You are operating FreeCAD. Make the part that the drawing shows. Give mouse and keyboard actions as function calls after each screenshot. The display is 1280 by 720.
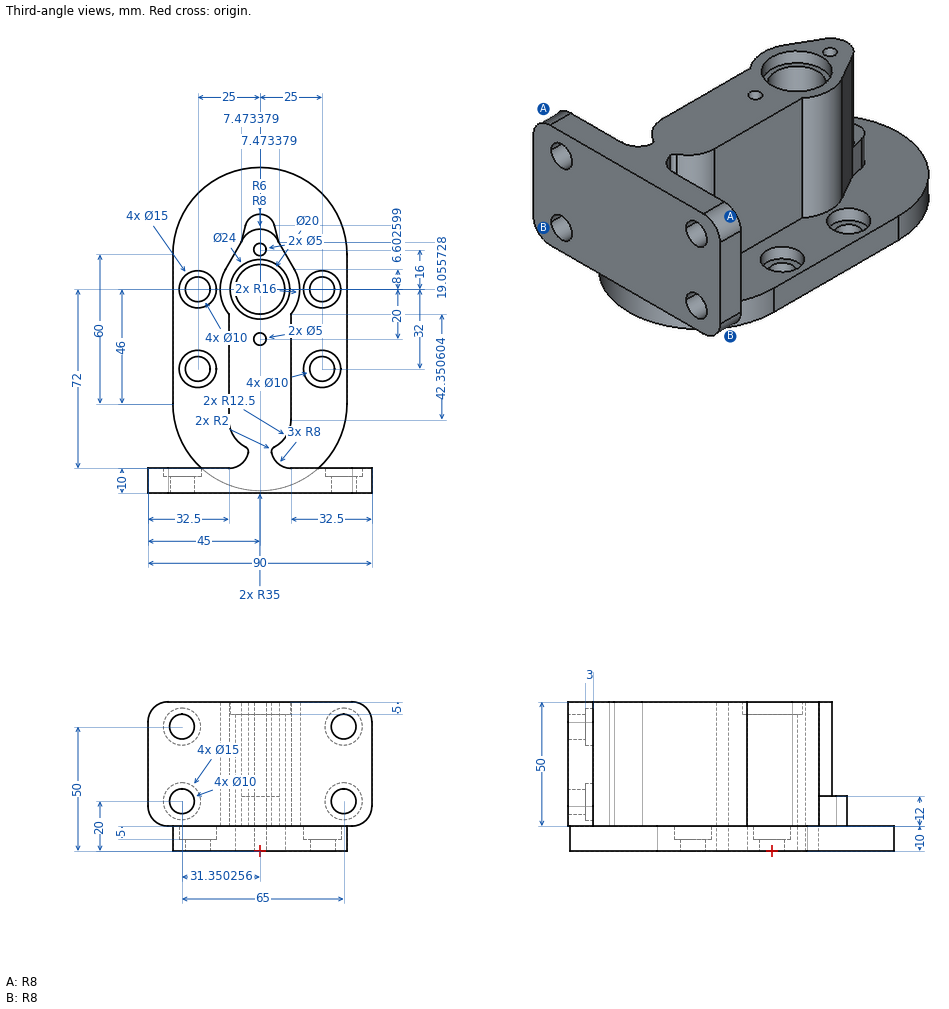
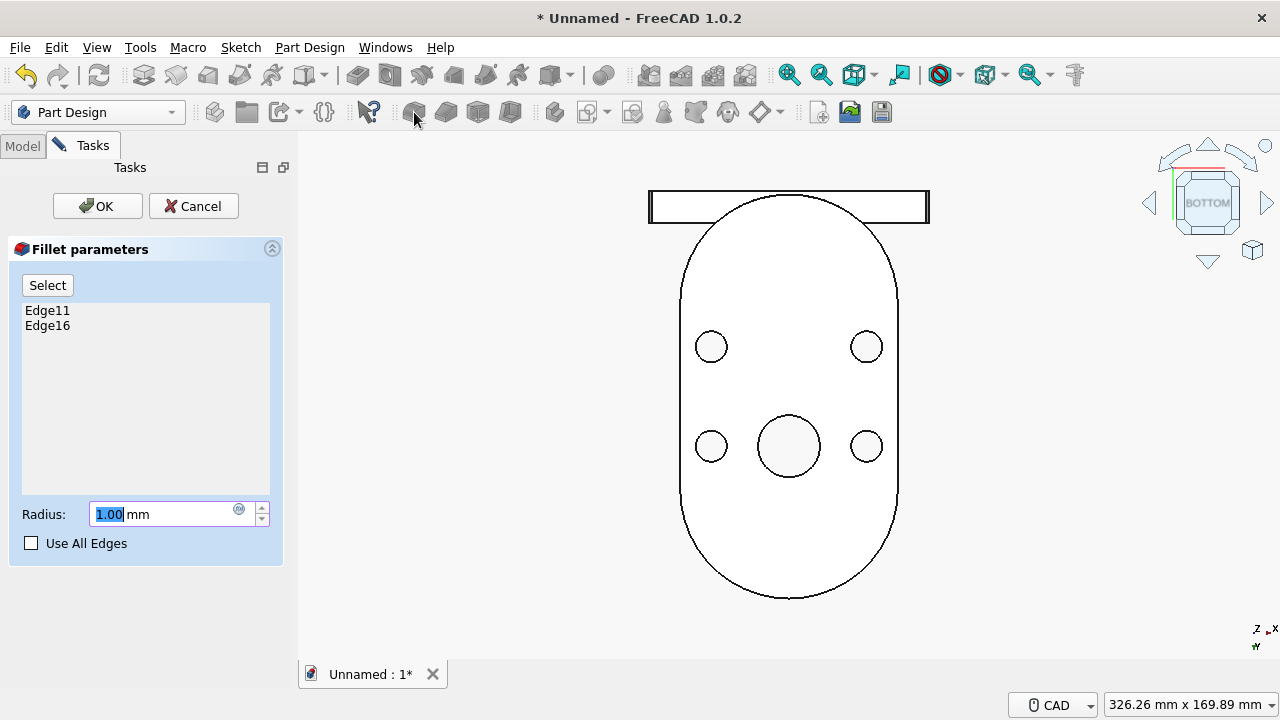
text(8)
key(Tab)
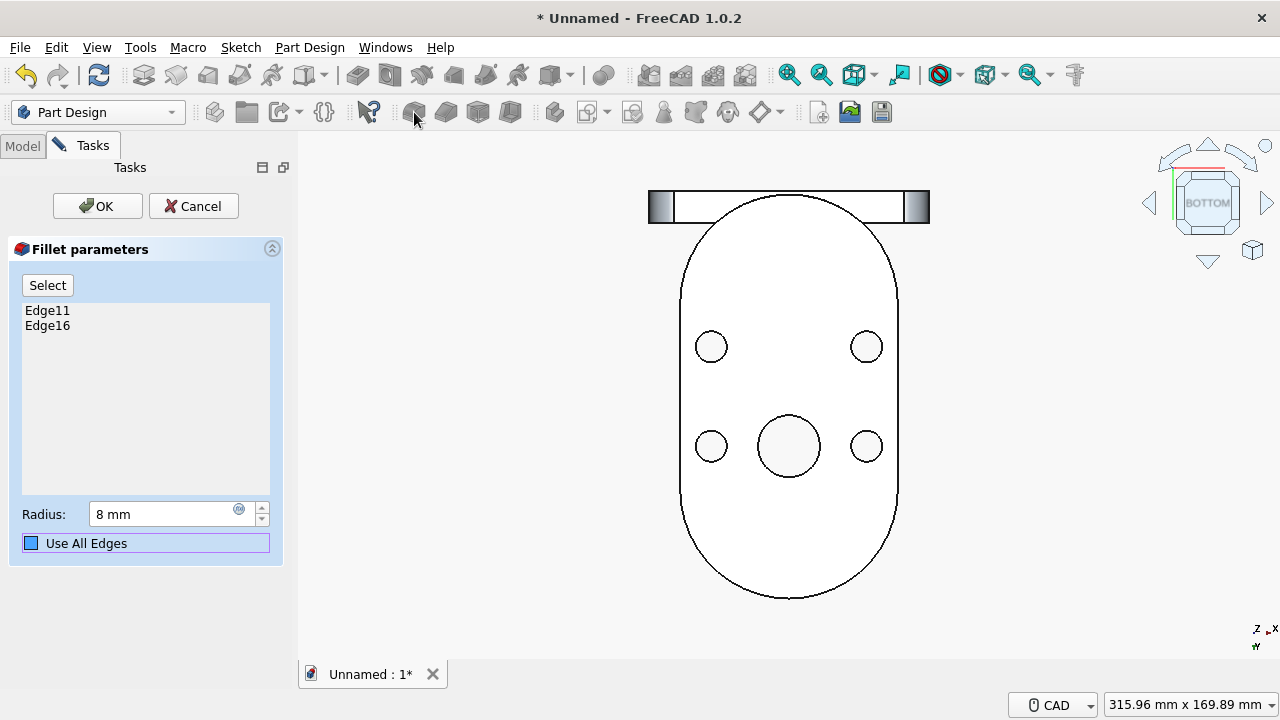
click(98, 206)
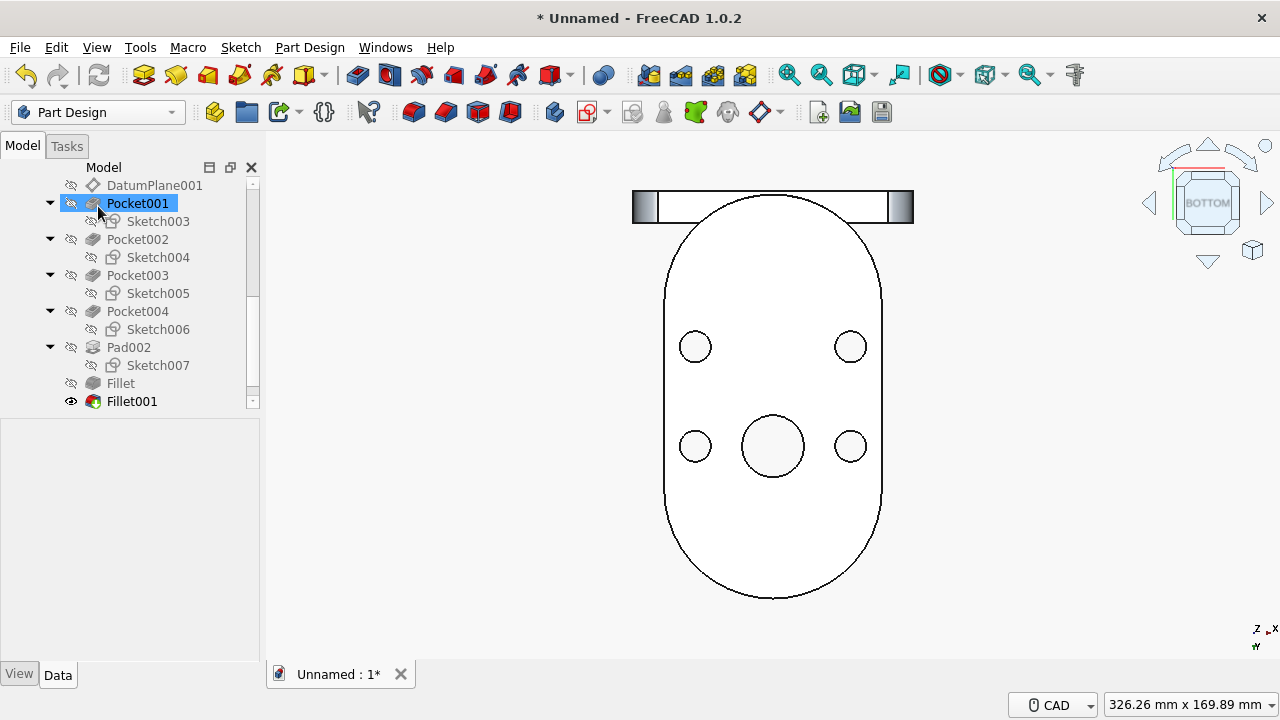
key(0)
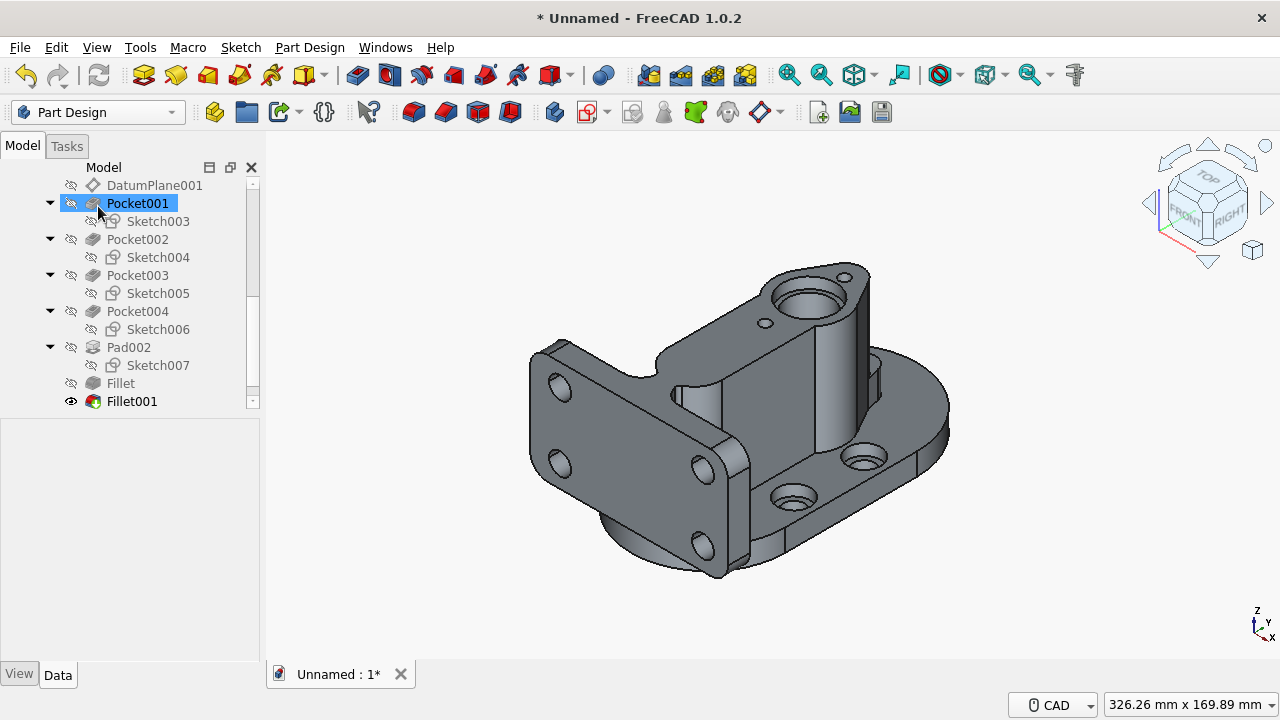
click(712, 353)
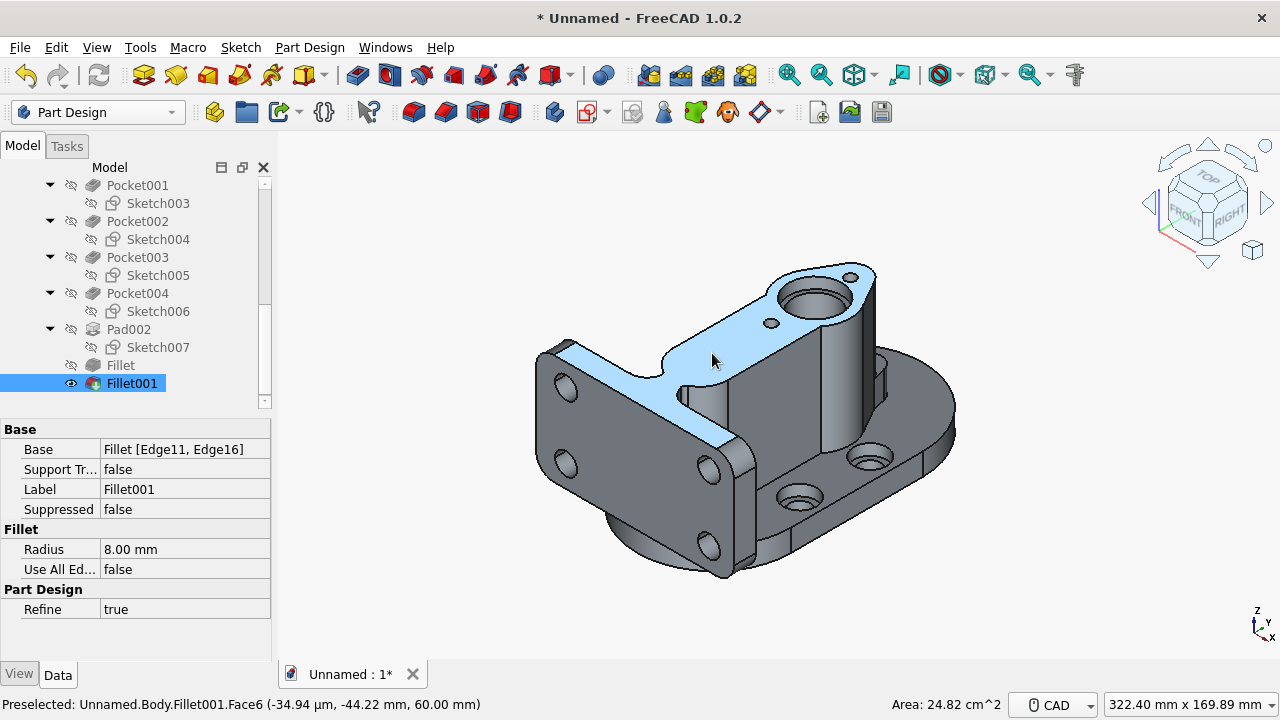
click(588, 112)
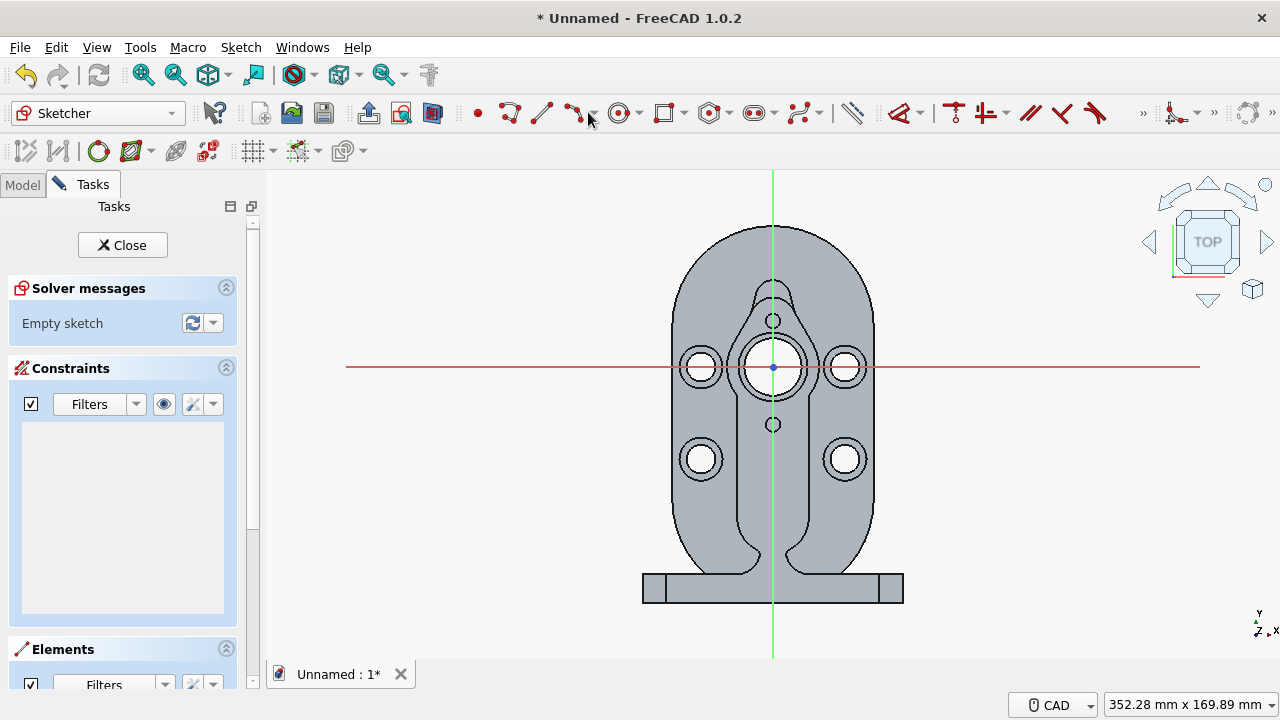
scroll(813, 348, up, 5)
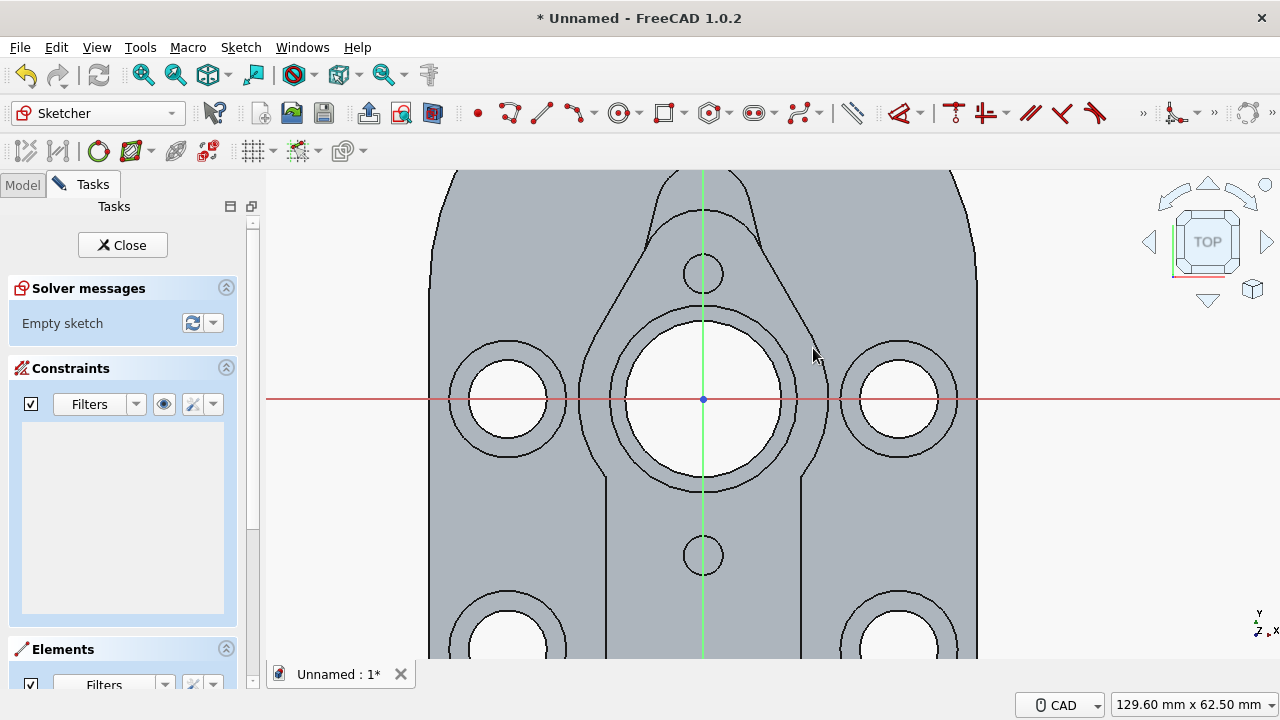
click(620, 114)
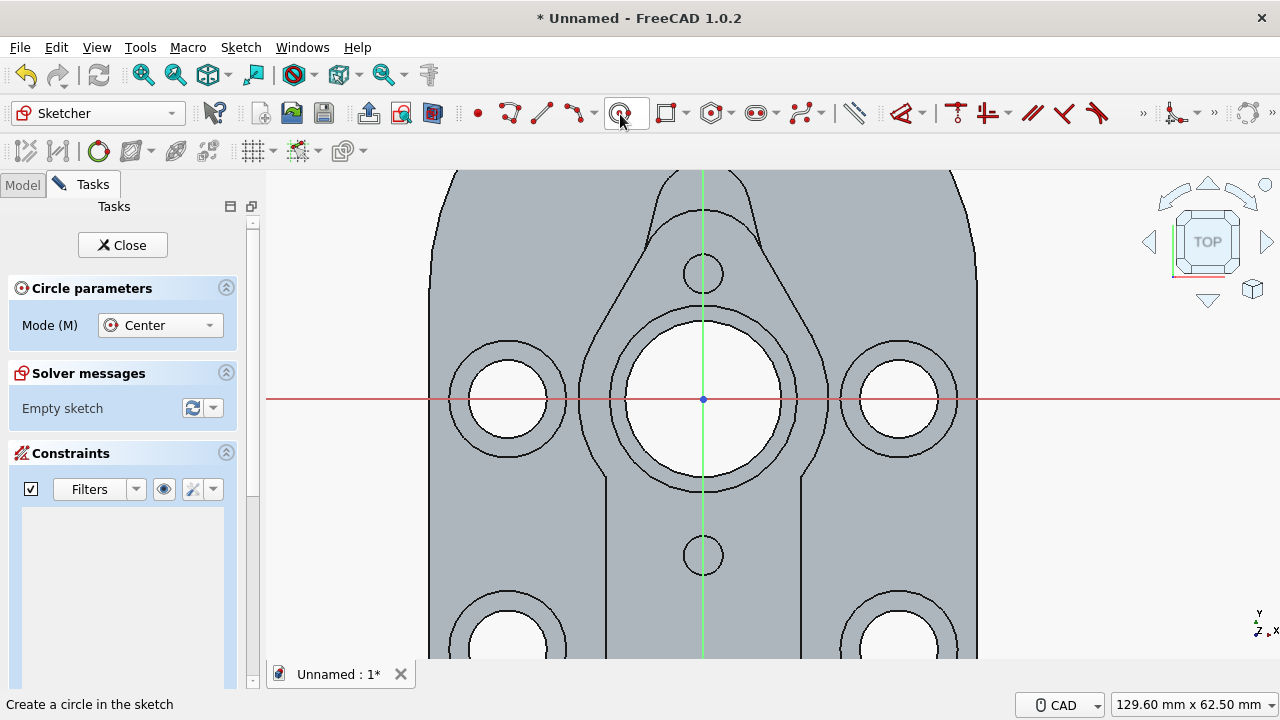
click(703, 274)
click(722, 267)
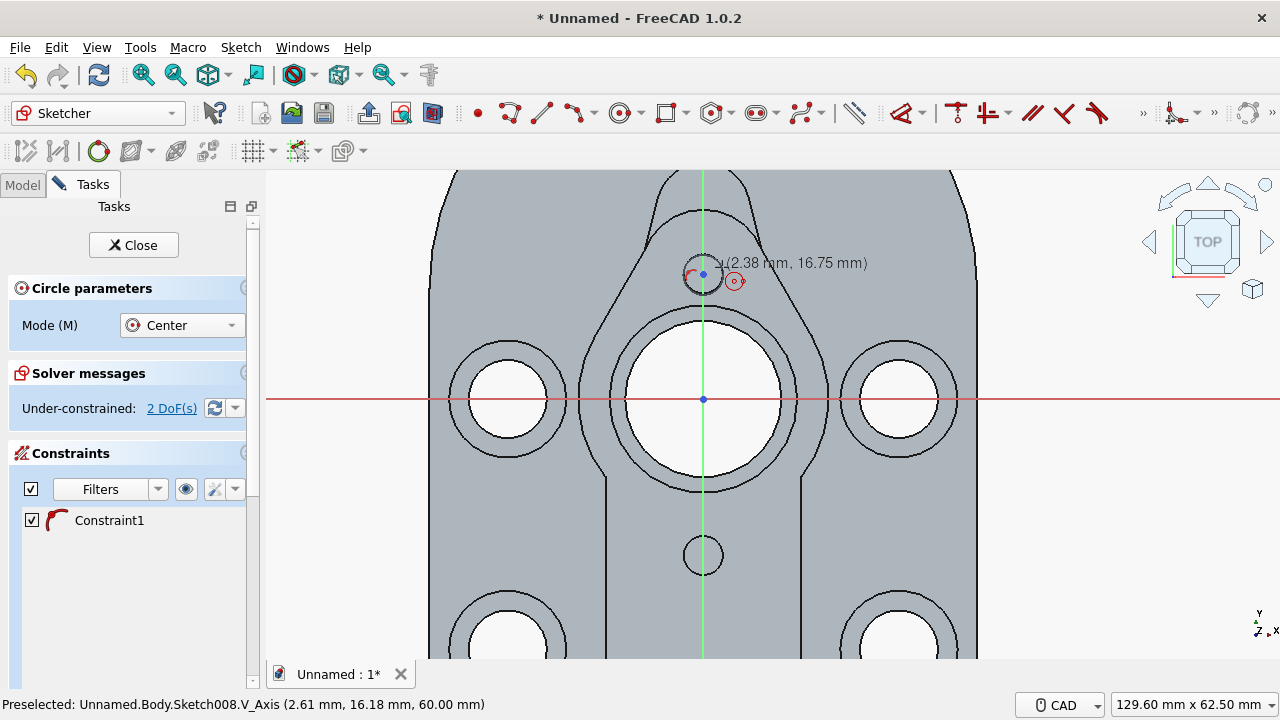
click(703, 556)
click(722, 549)
key(Escape)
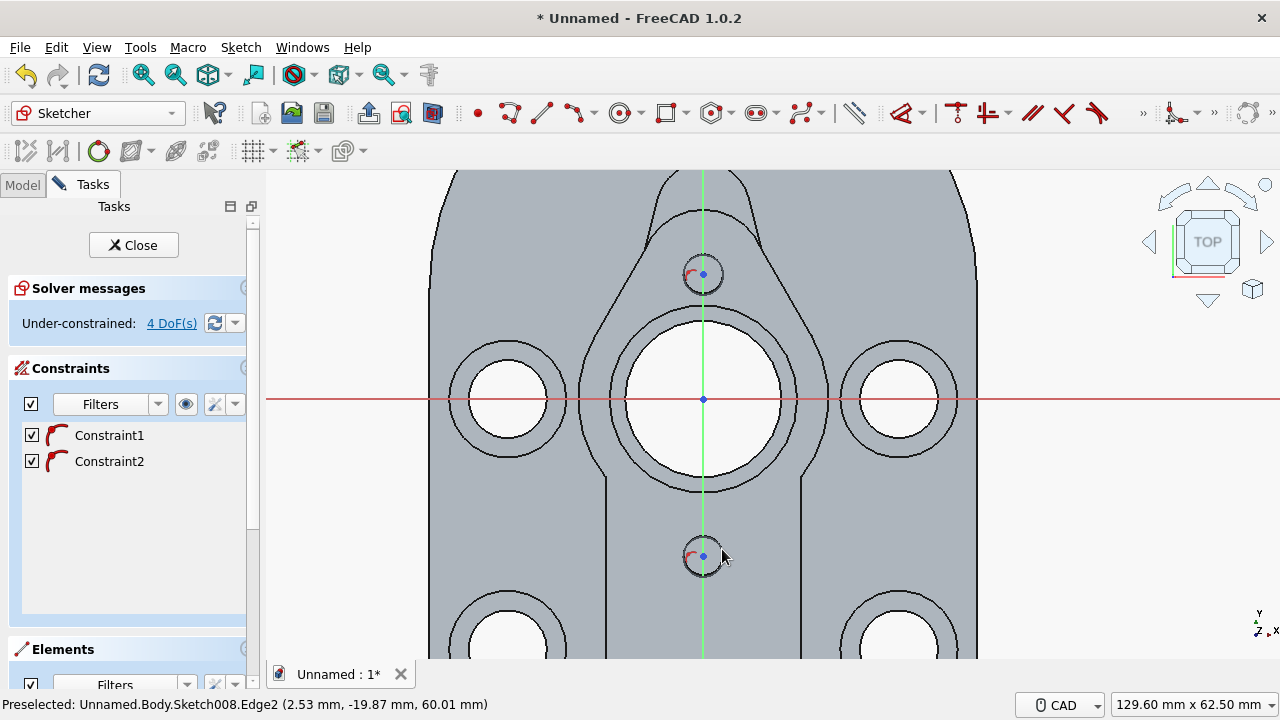
click(717, 261)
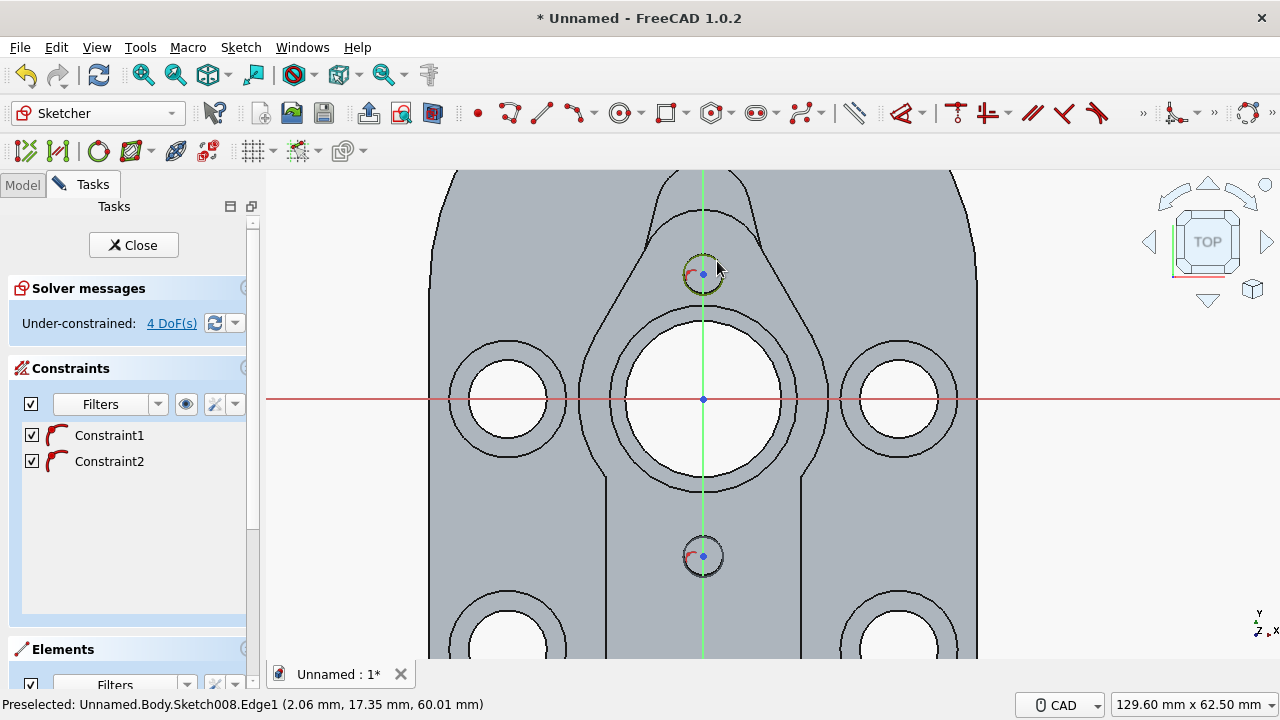
click(717, 543)